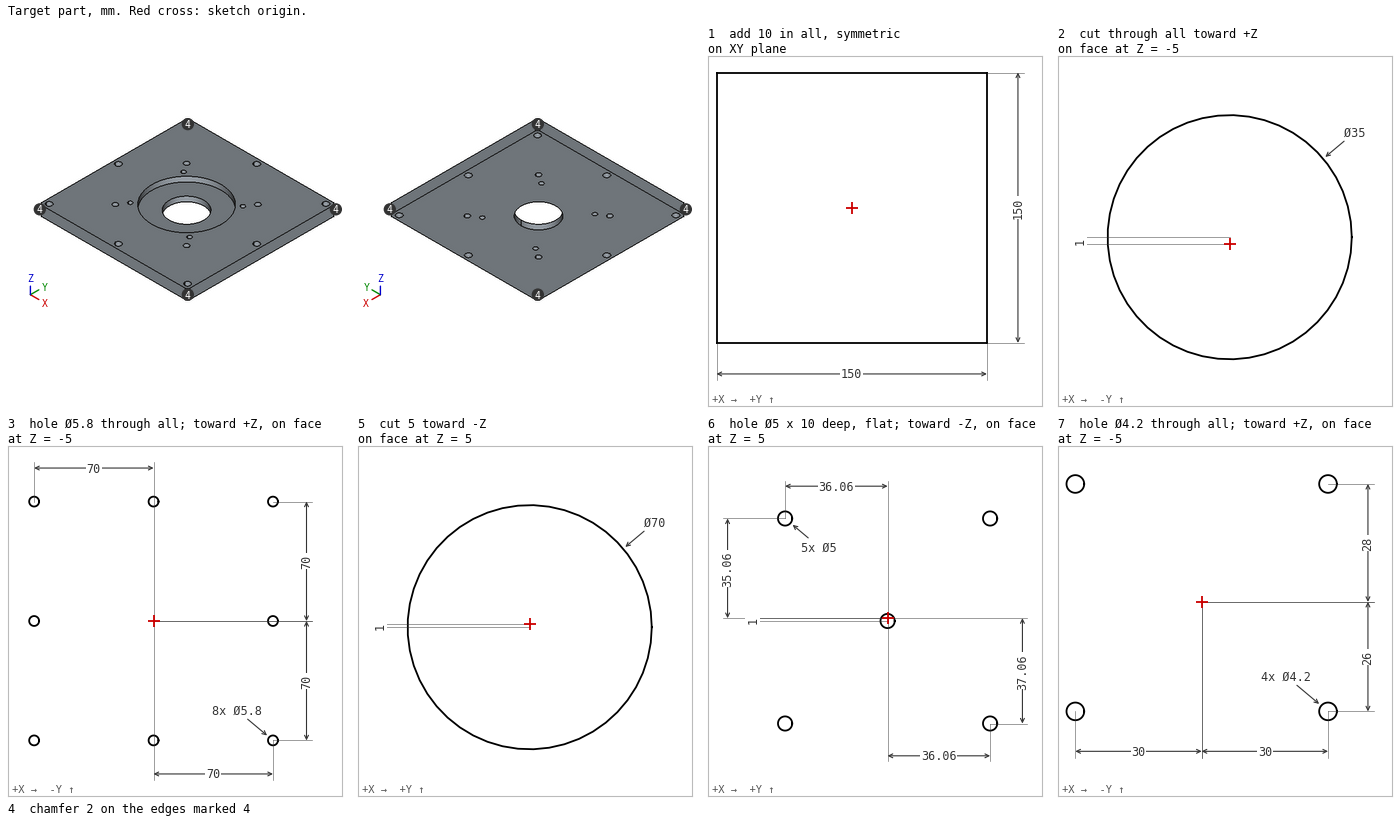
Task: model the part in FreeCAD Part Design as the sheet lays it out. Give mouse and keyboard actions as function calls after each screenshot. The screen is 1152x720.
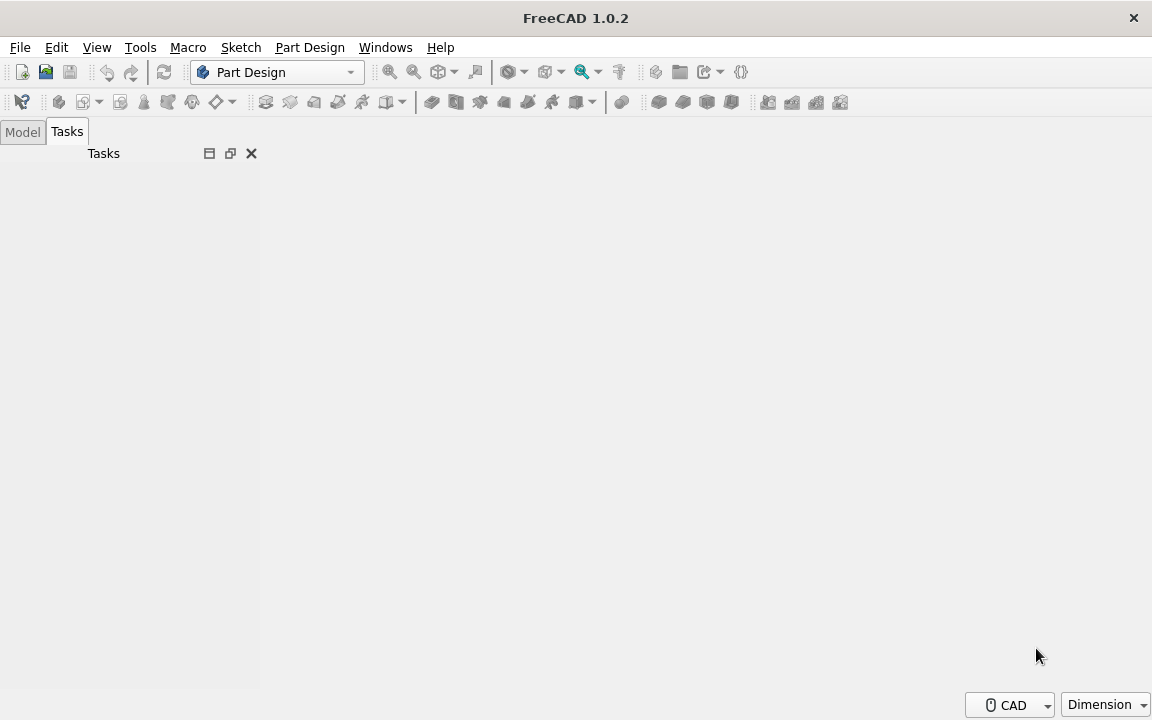
key(ctrl+n)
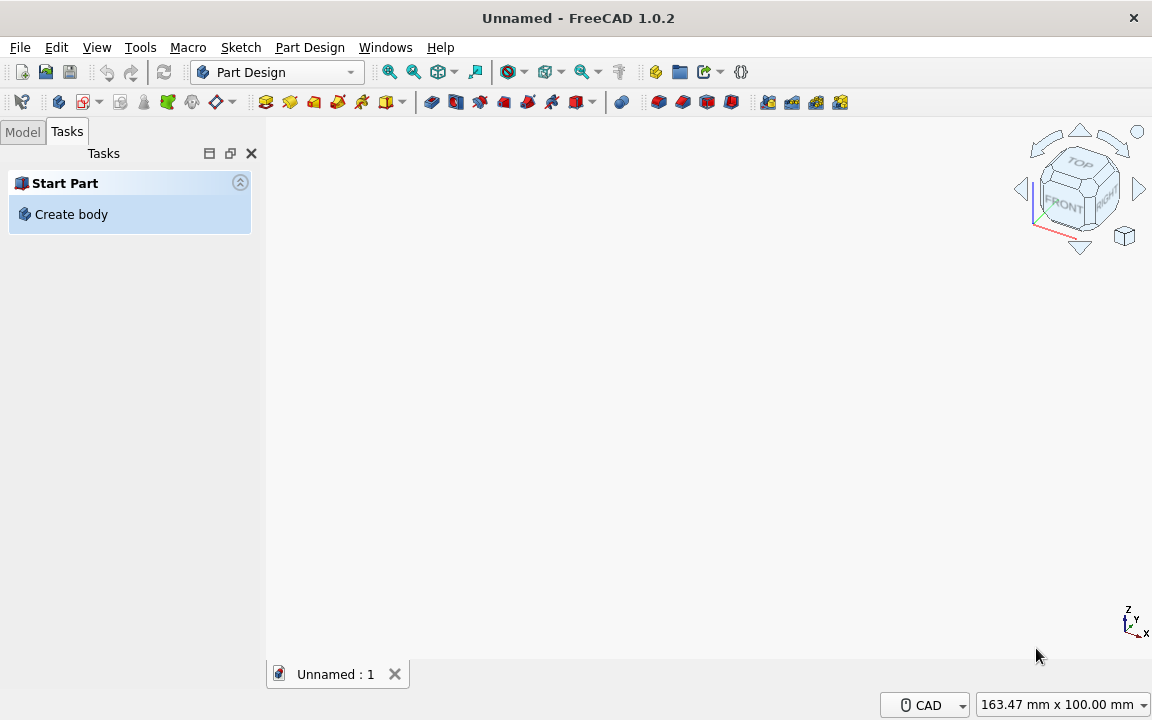
click(84, 102)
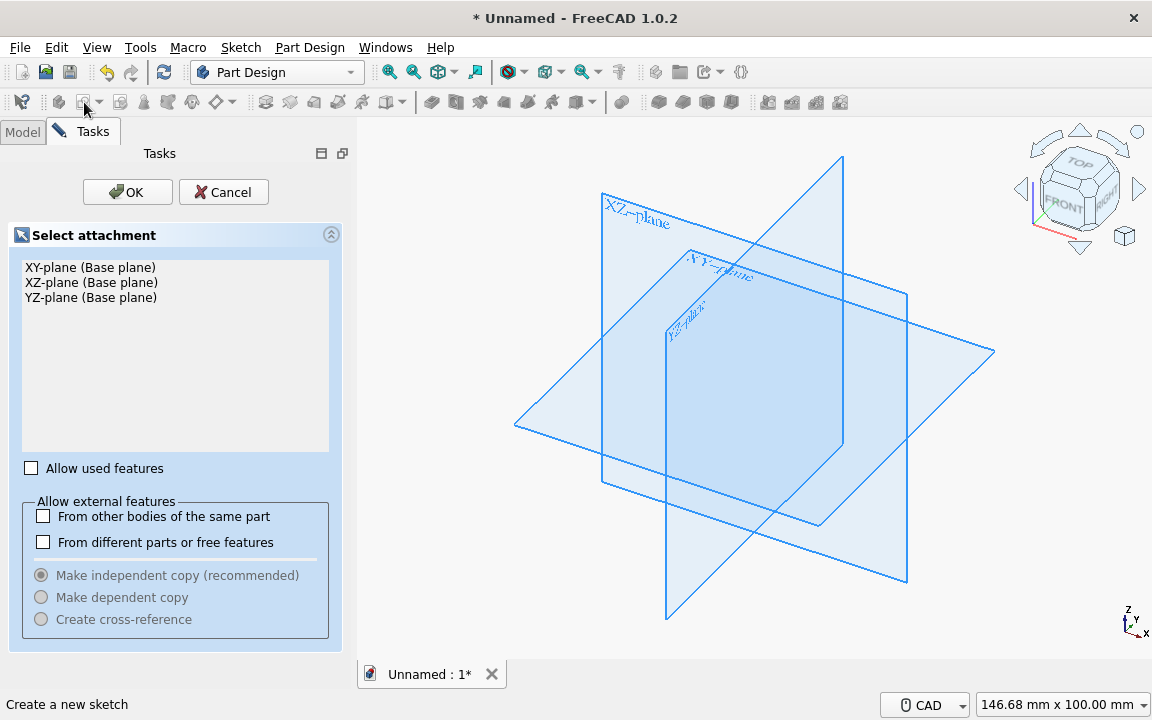
click(82, 268)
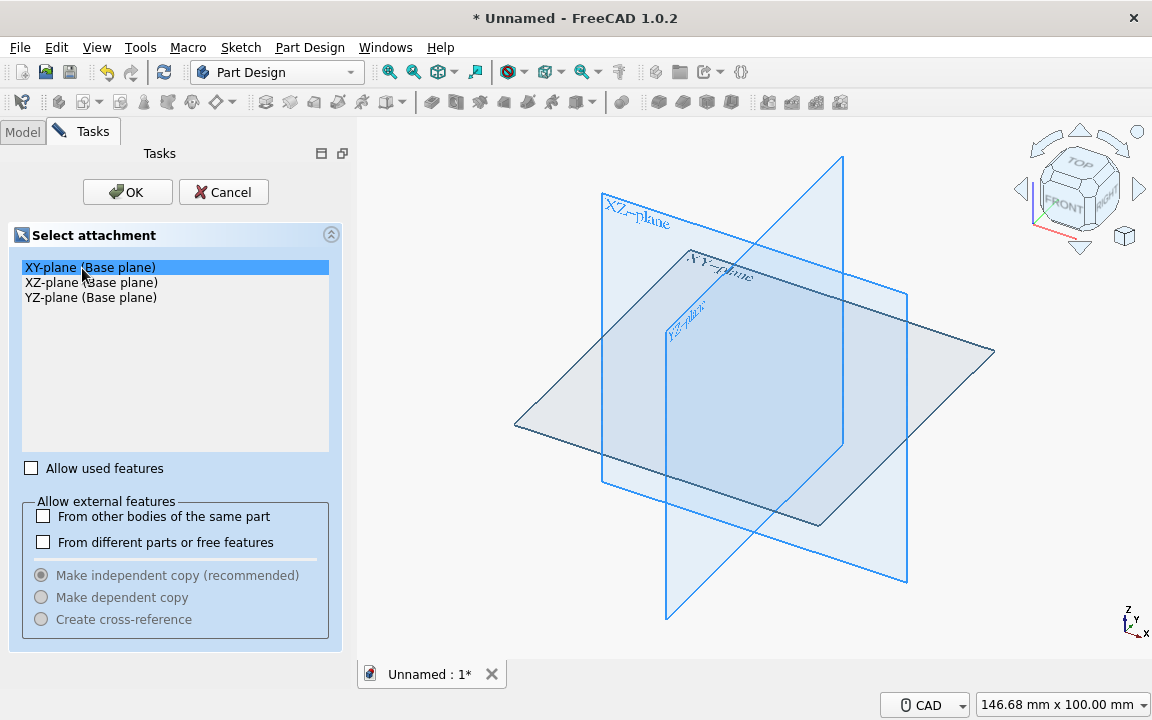
click(128, 192)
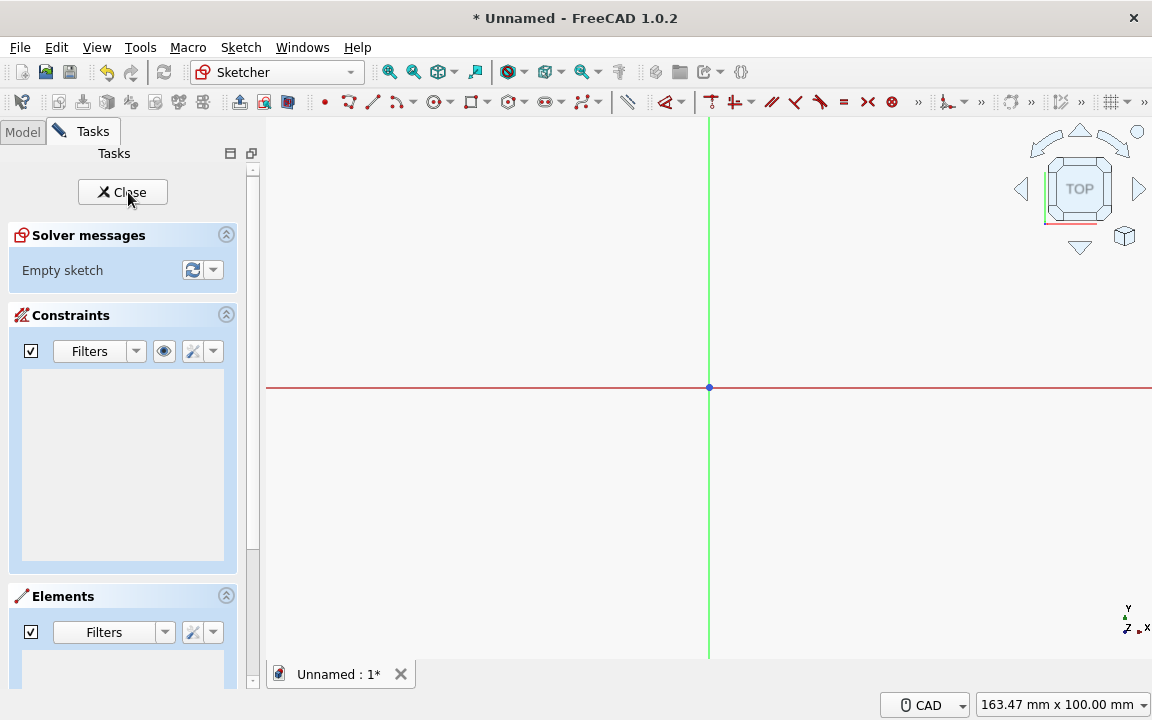
scroll(585, 388, down, 4)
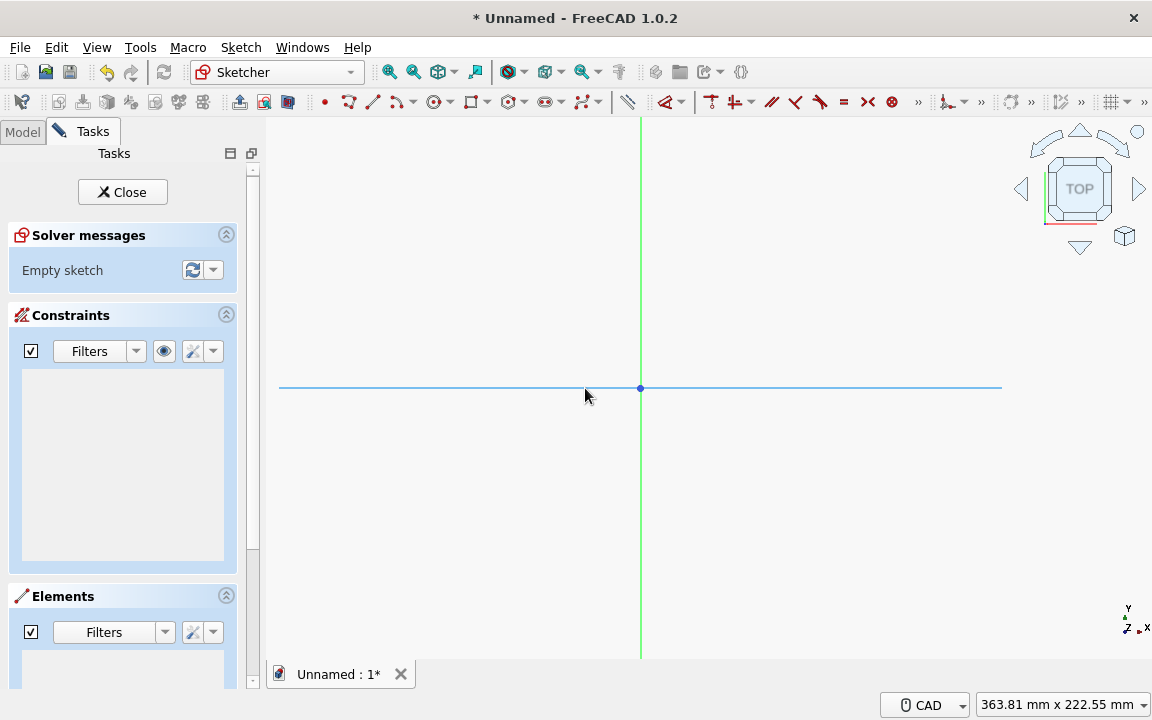
click(490, 102)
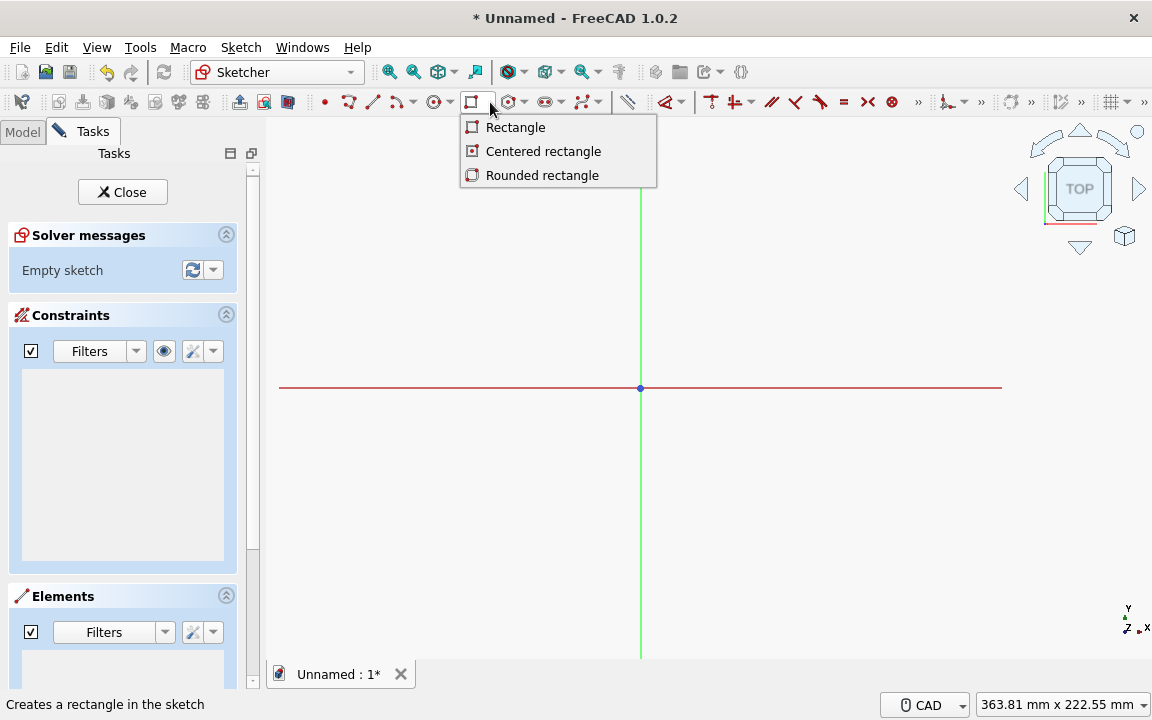
click(558, 151)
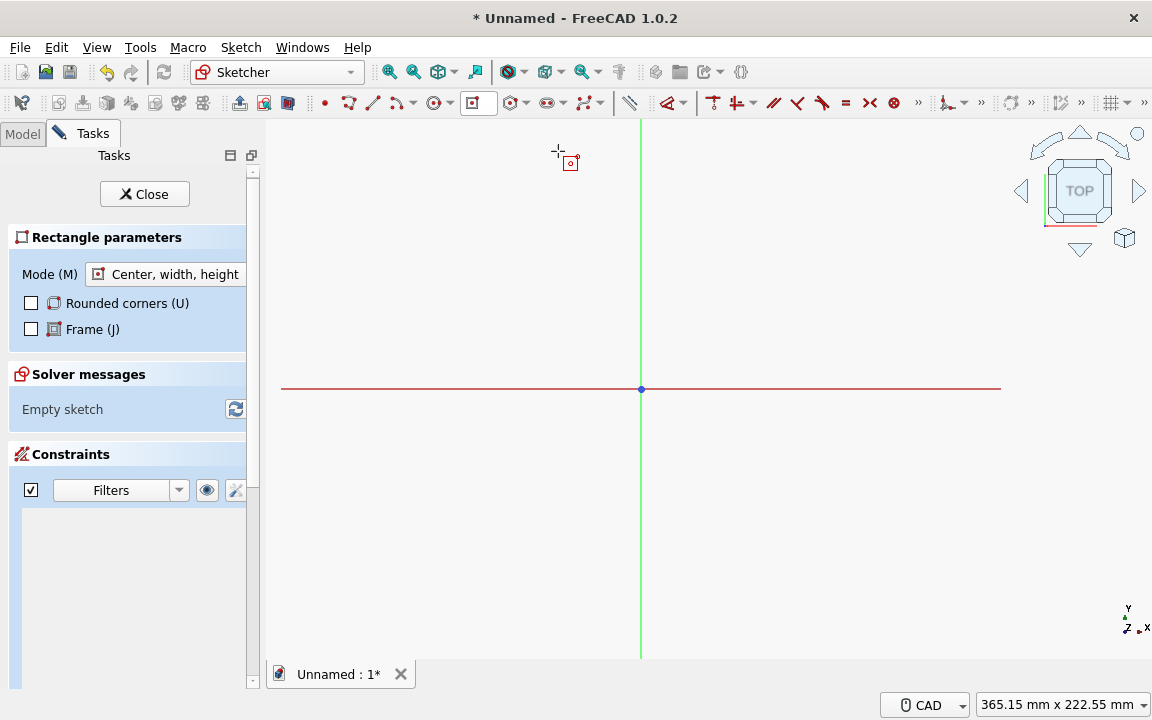
click(641, 389)
move(823, 207)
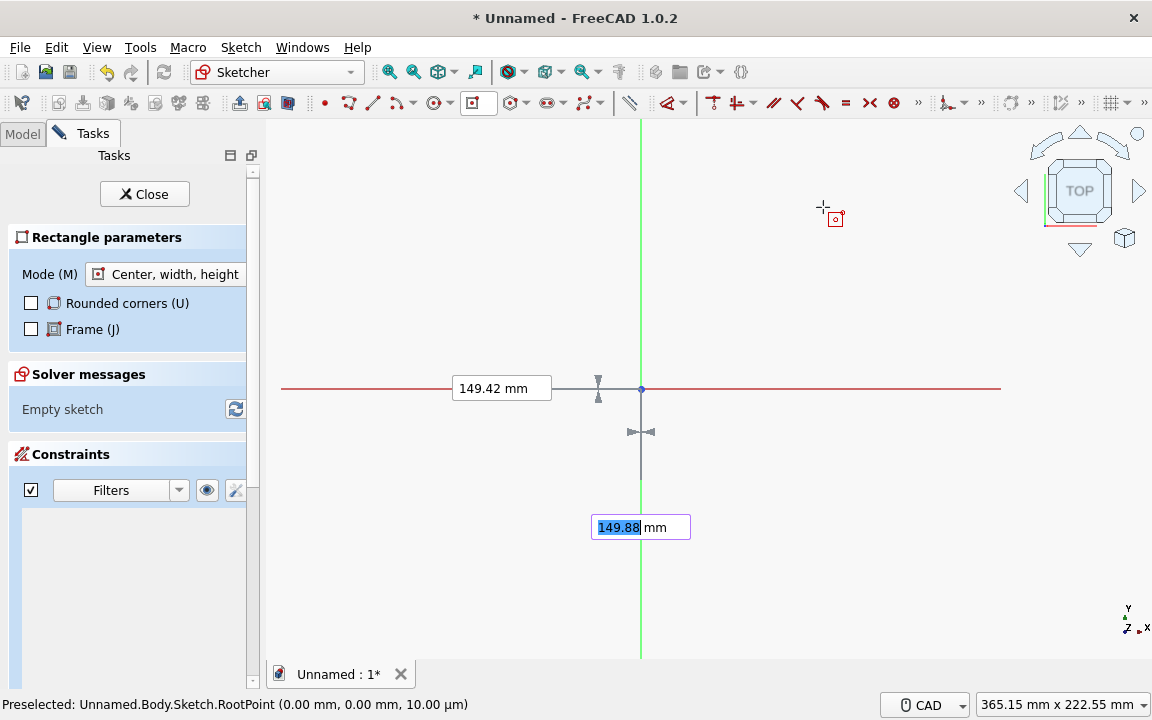
text(150)
key(Tab)
text(150)
key(Return)
key(Escape)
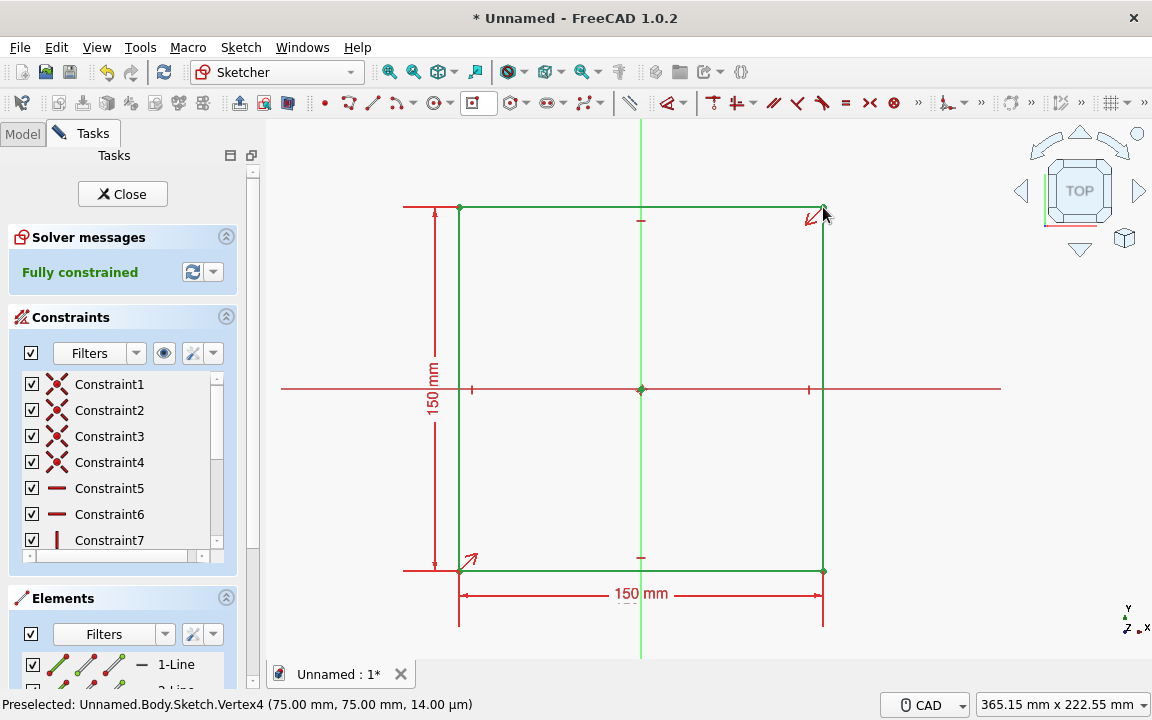
click(123, 194)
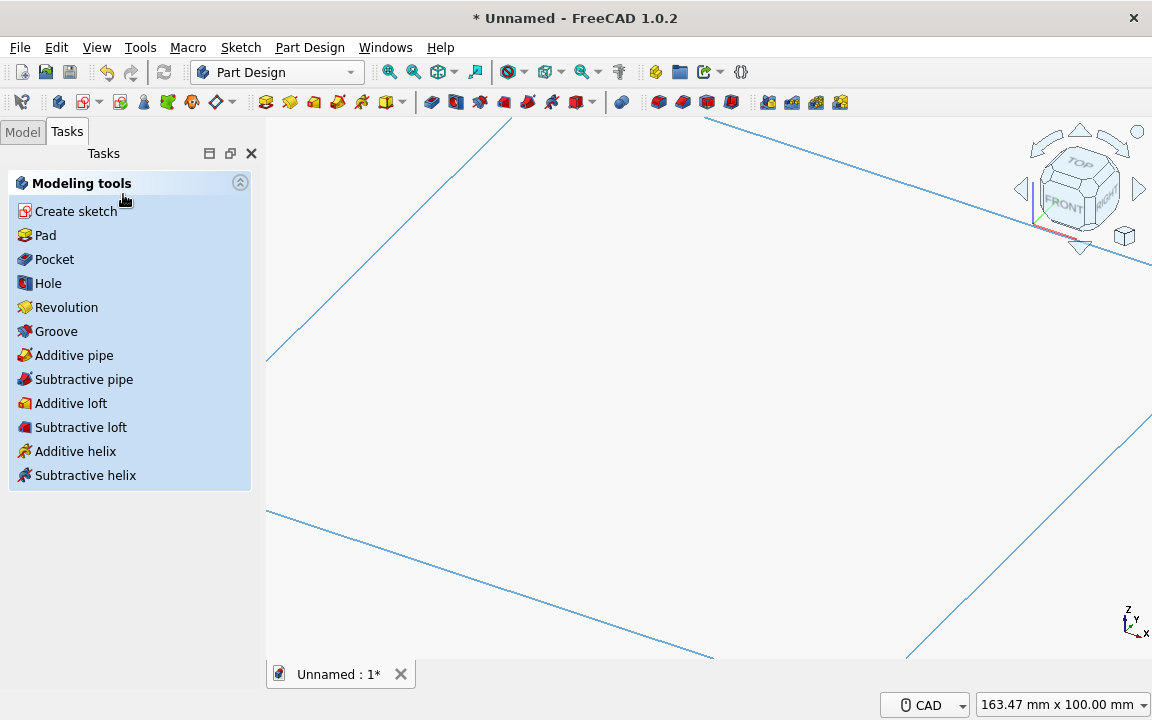
click(266, 102)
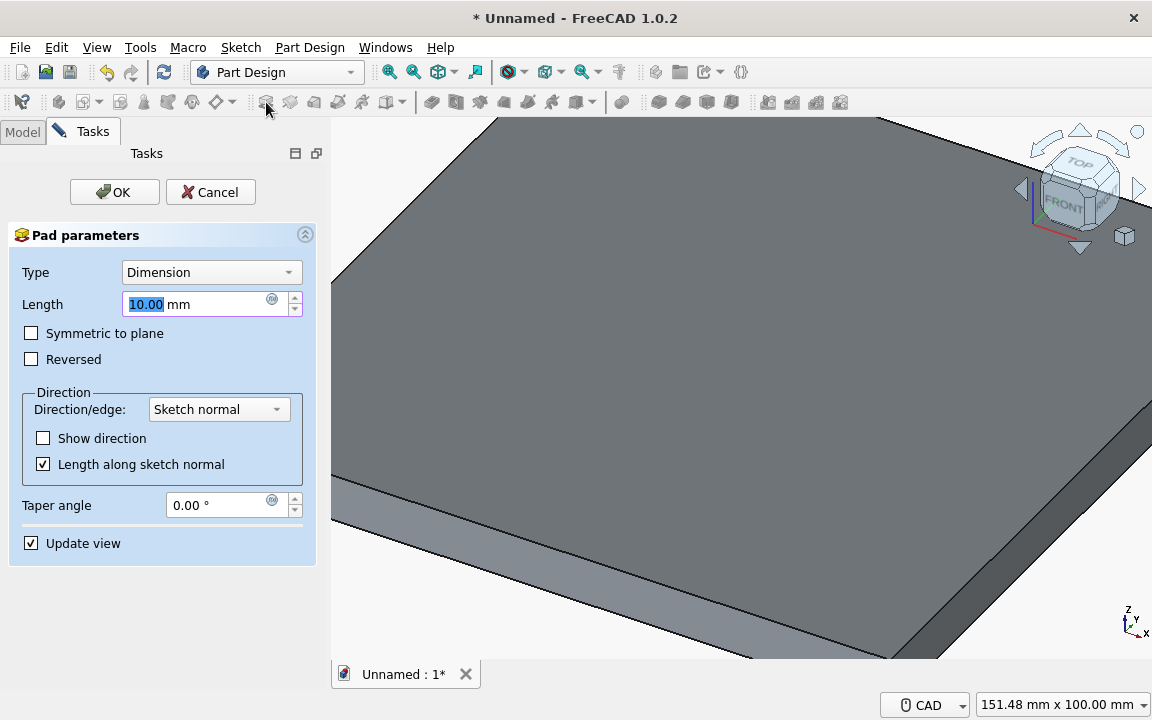
text(10)
key(Tab)